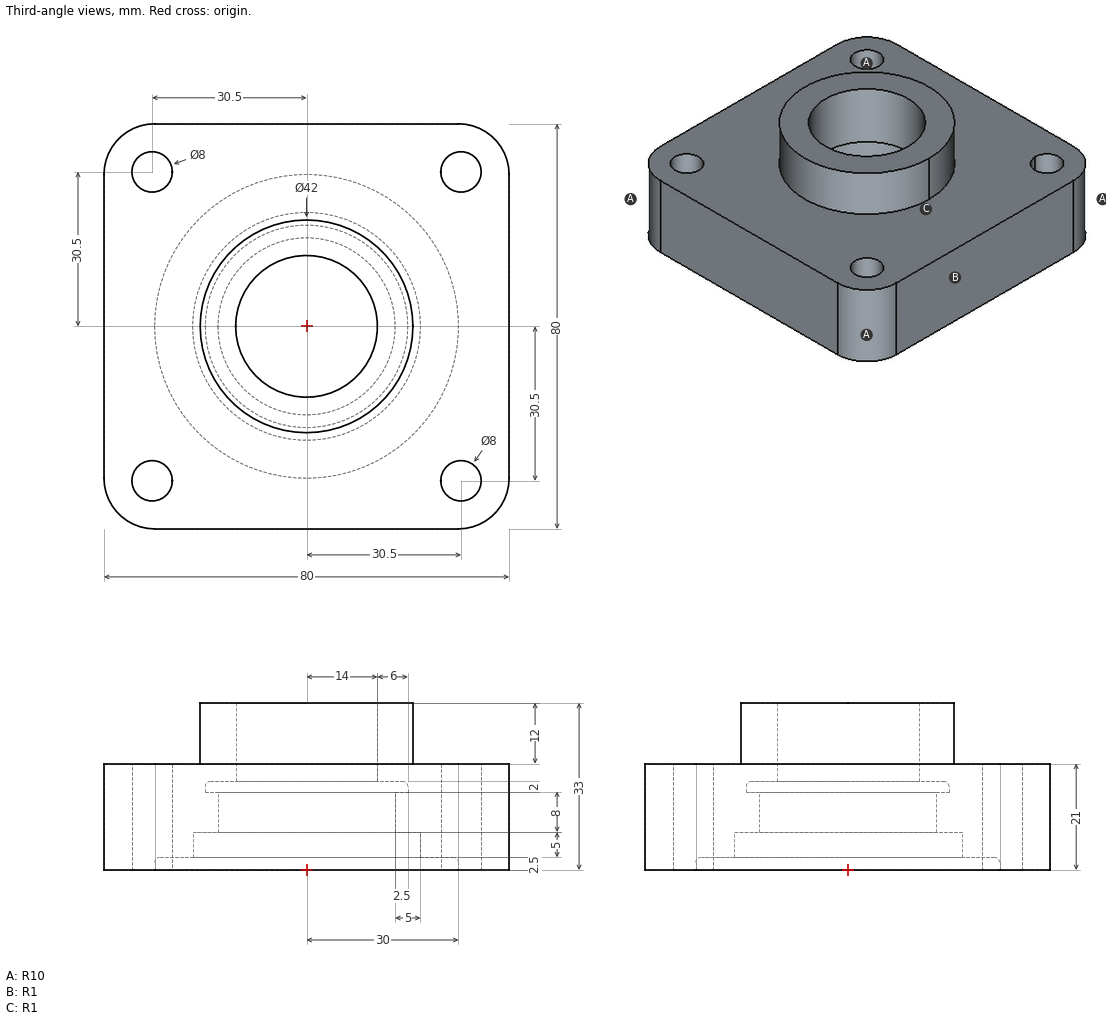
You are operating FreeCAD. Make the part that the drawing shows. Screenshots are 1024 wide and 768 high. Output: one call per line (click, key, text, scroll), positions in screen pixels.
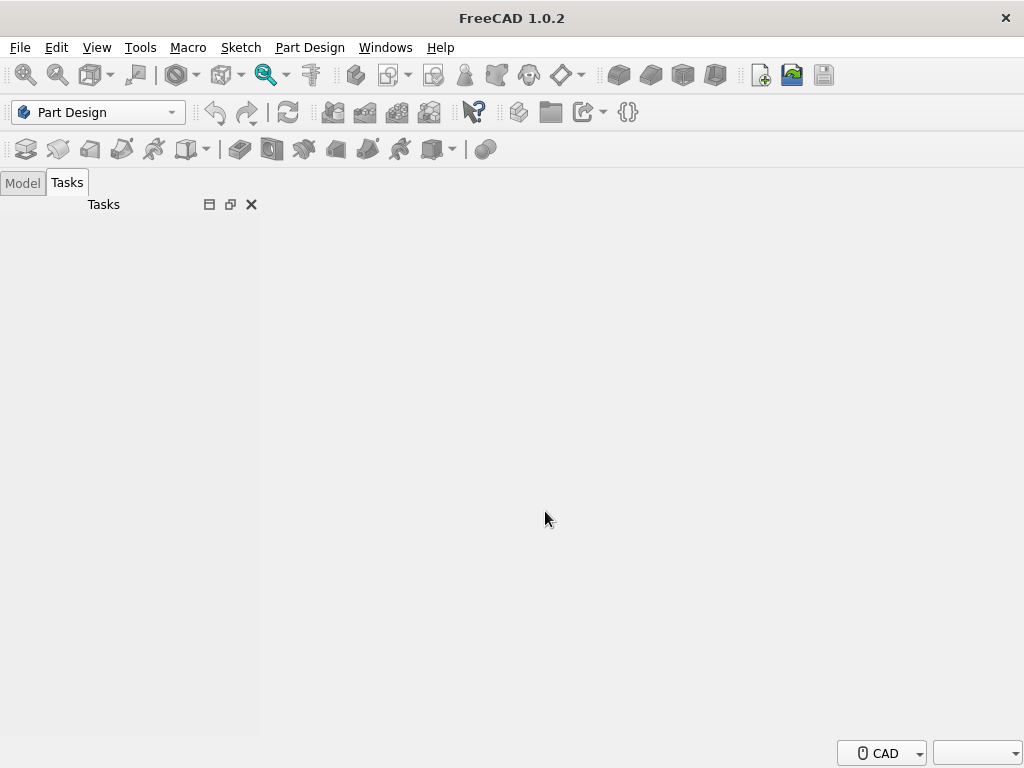
click(760, 76)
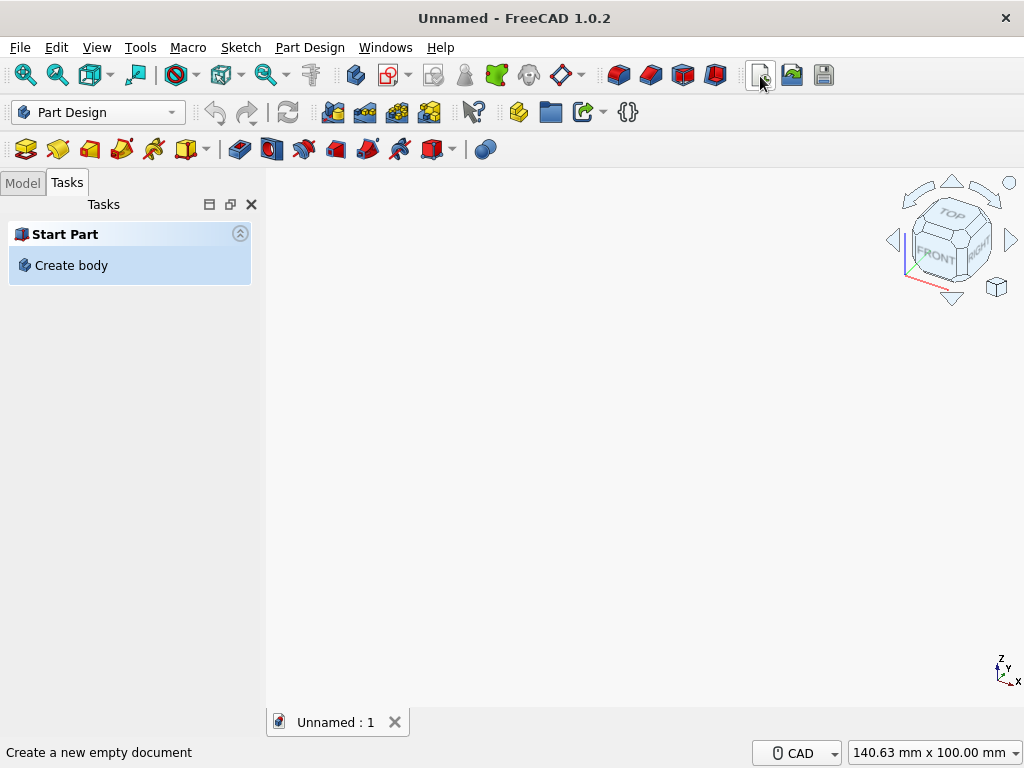
click(388, 76)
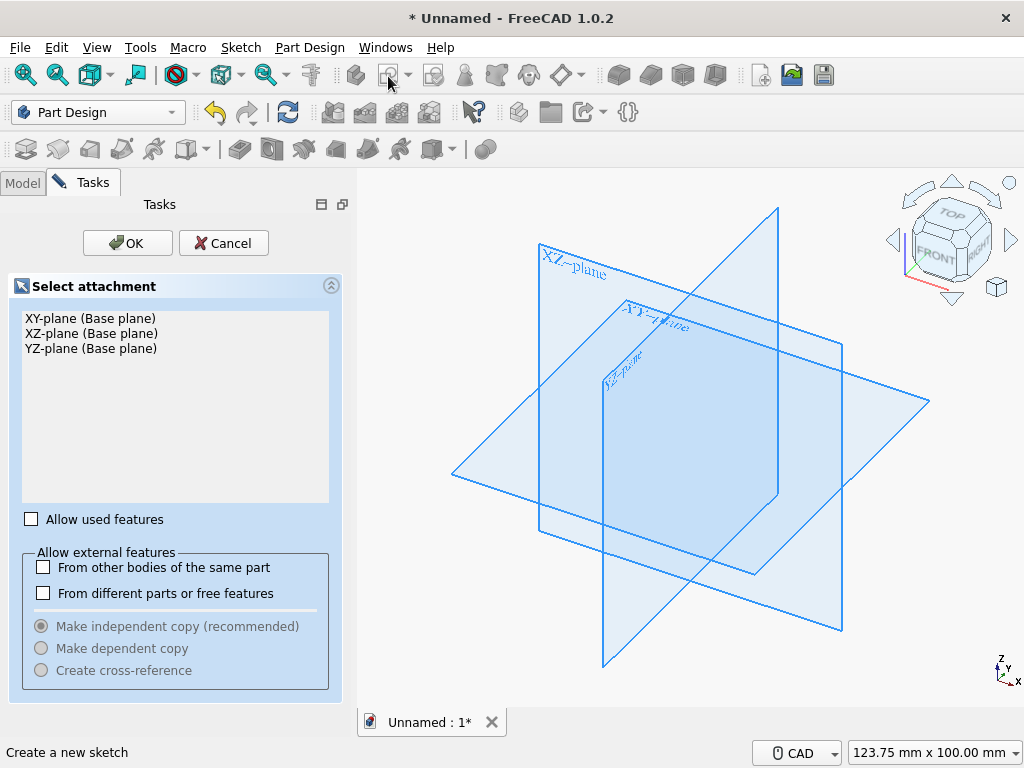
click(82, 318)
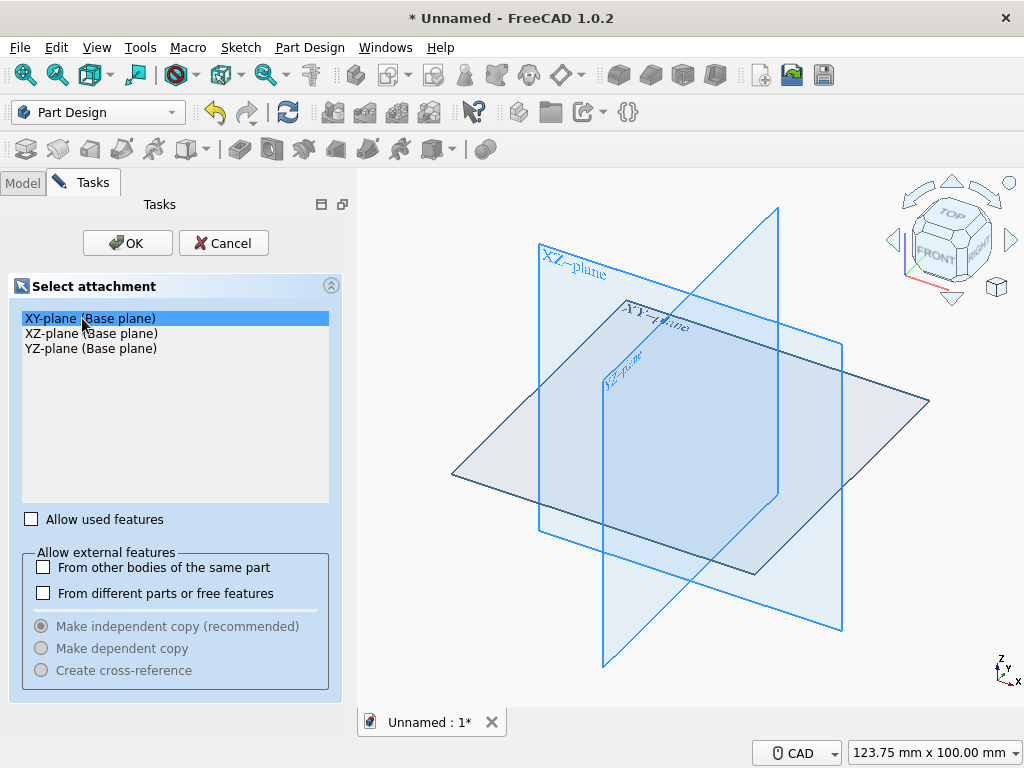
click(128, 243)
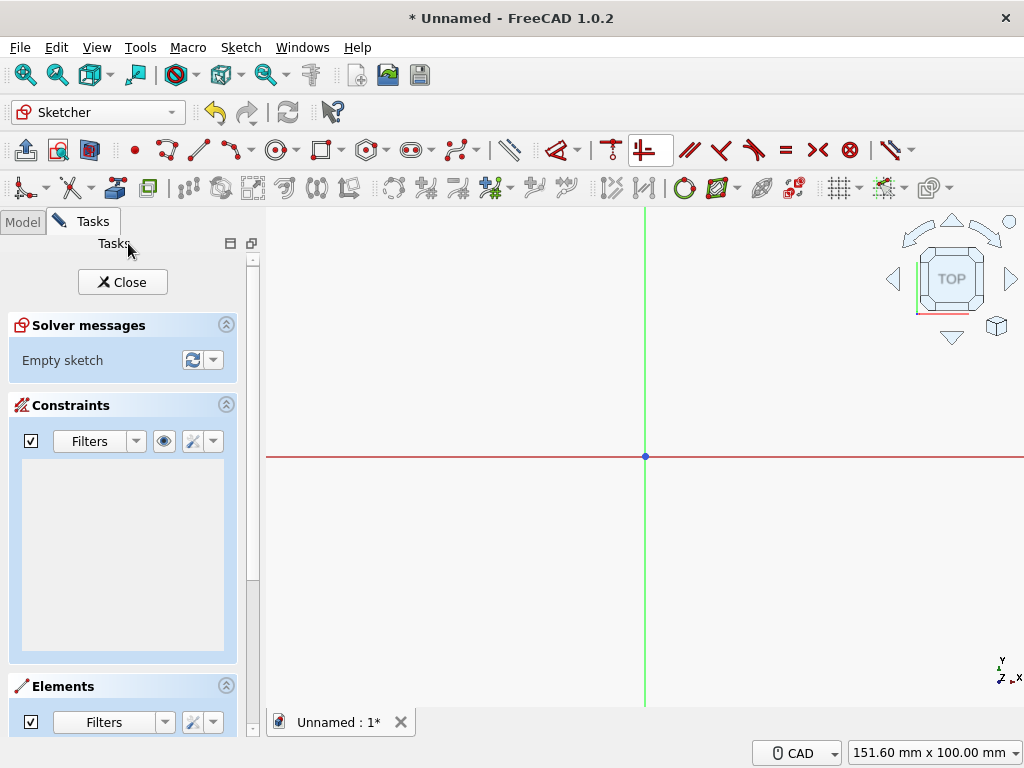
scroll(294, 457, down, 1)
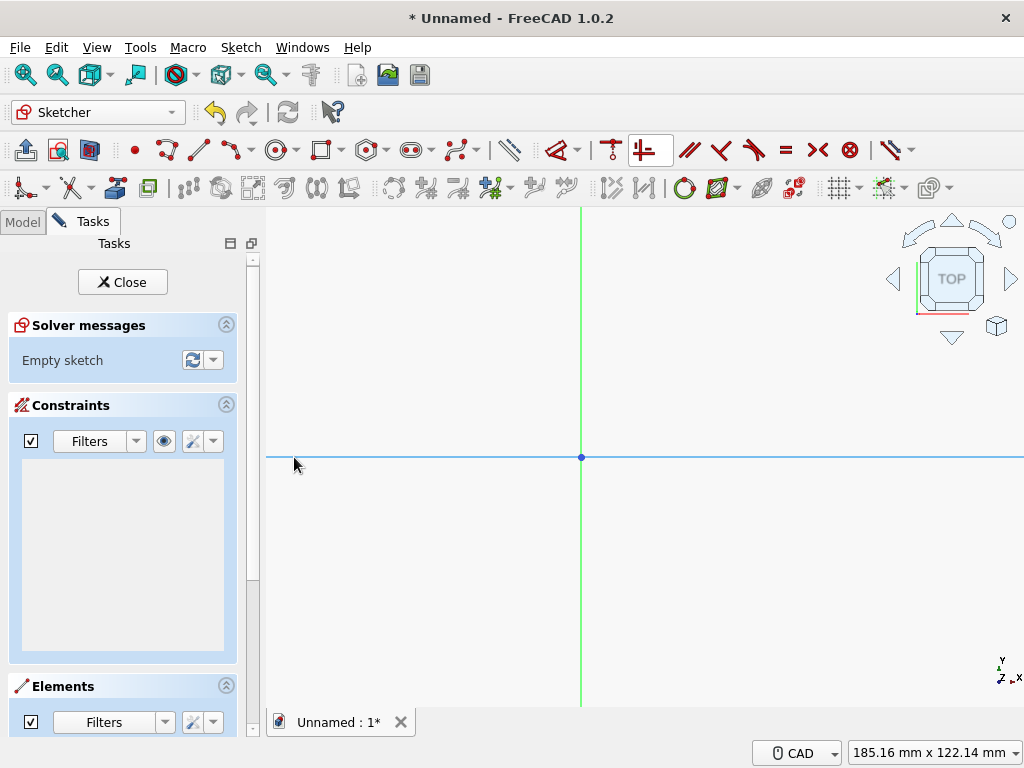
key(g)
key(v)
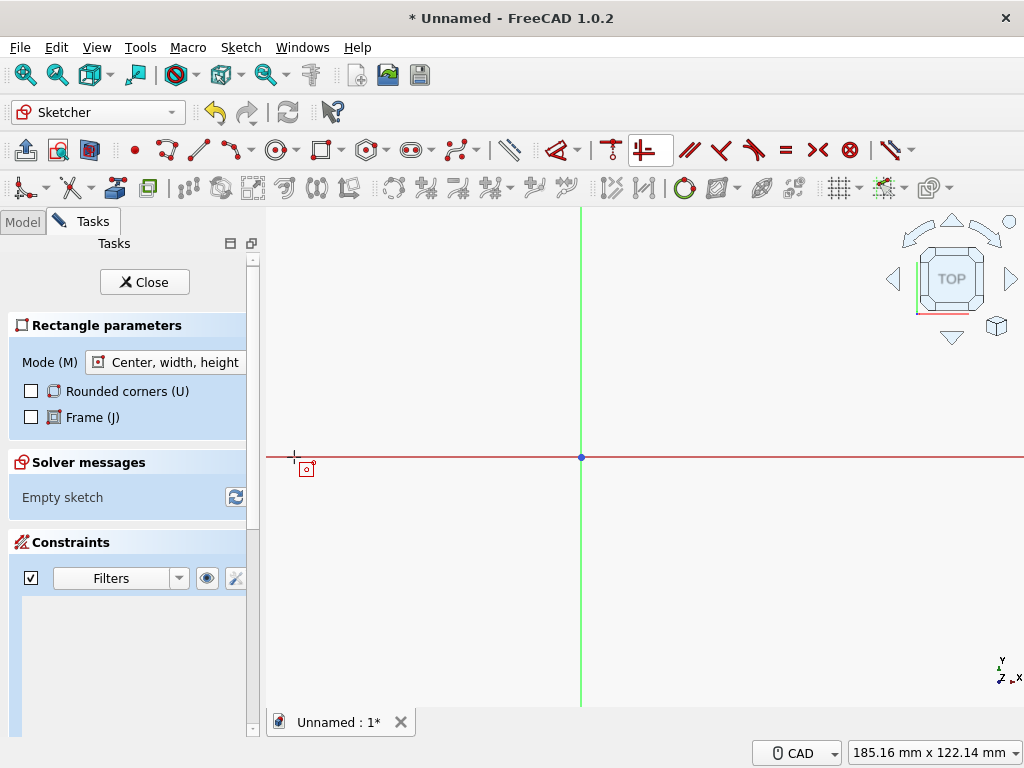
click(581, 457)
move(745, 293)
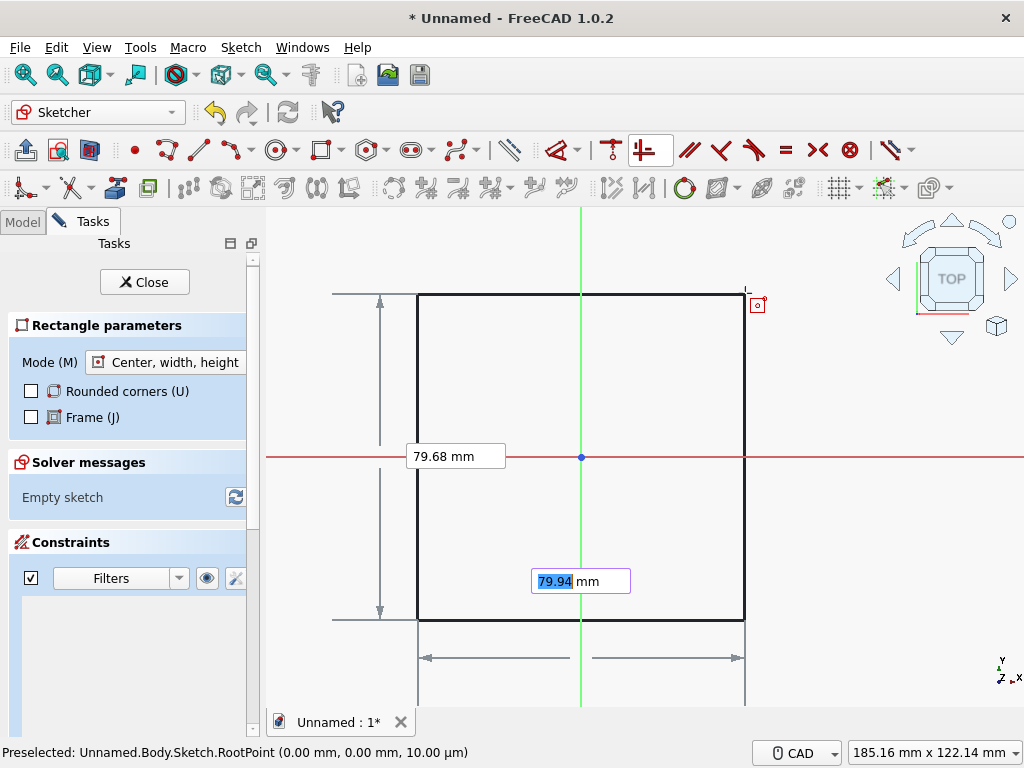
text(80)
key(Tab)
text(80)
key(Return)
key(Escape)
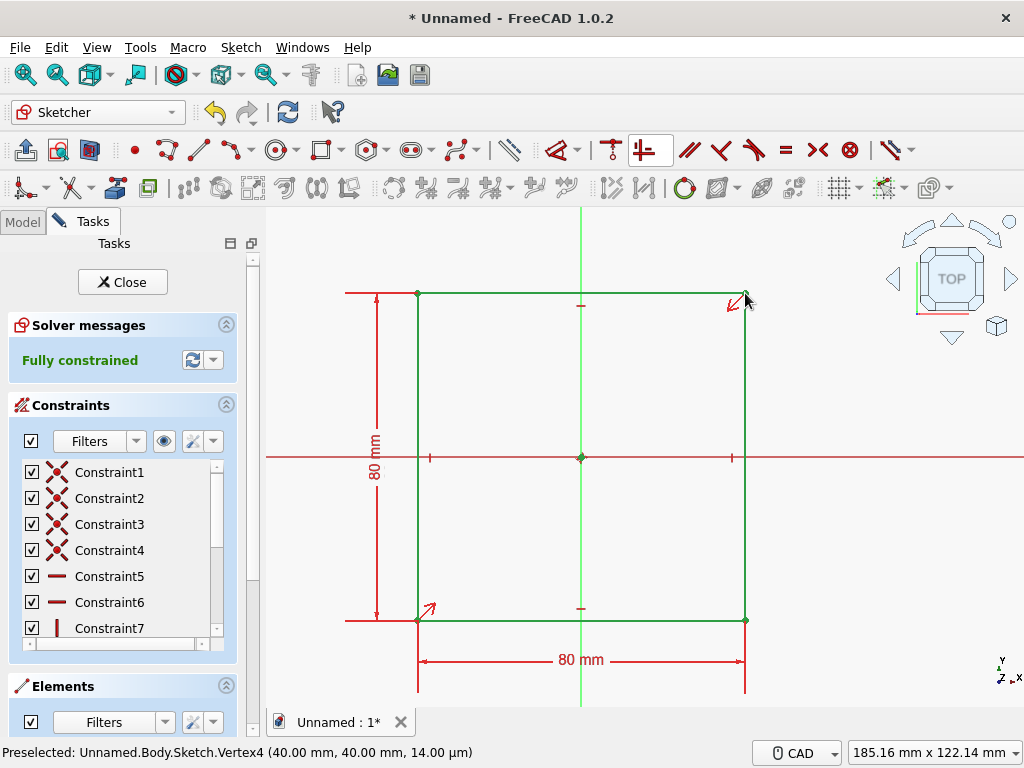
click(123, 282)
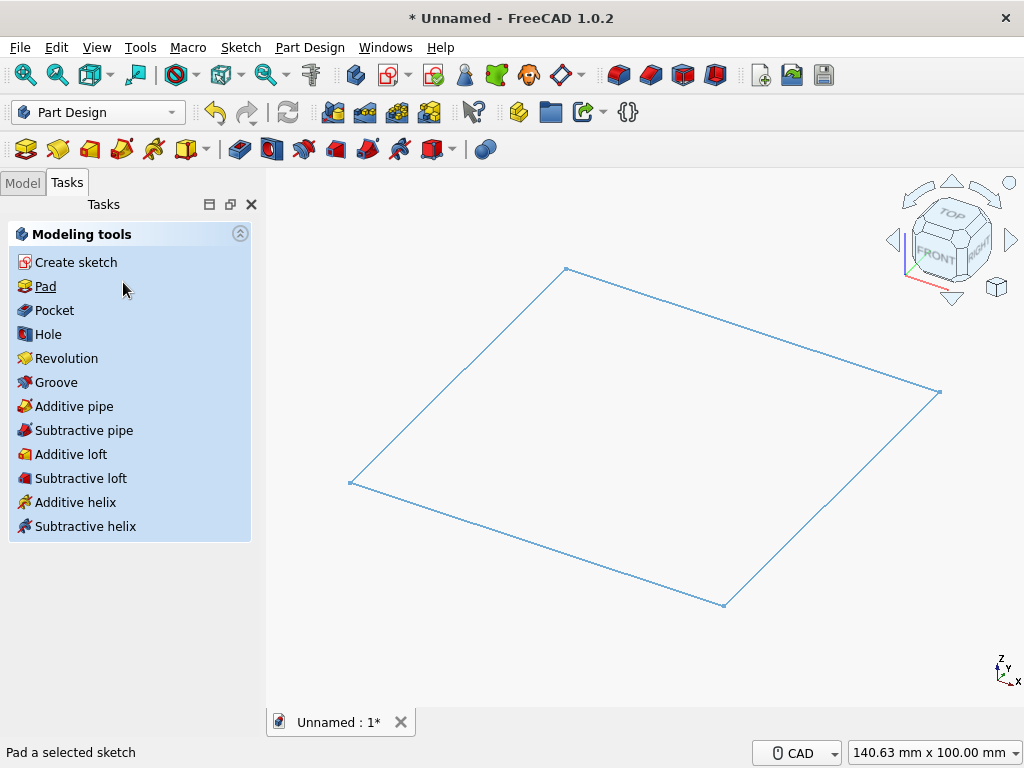
click(26, 150)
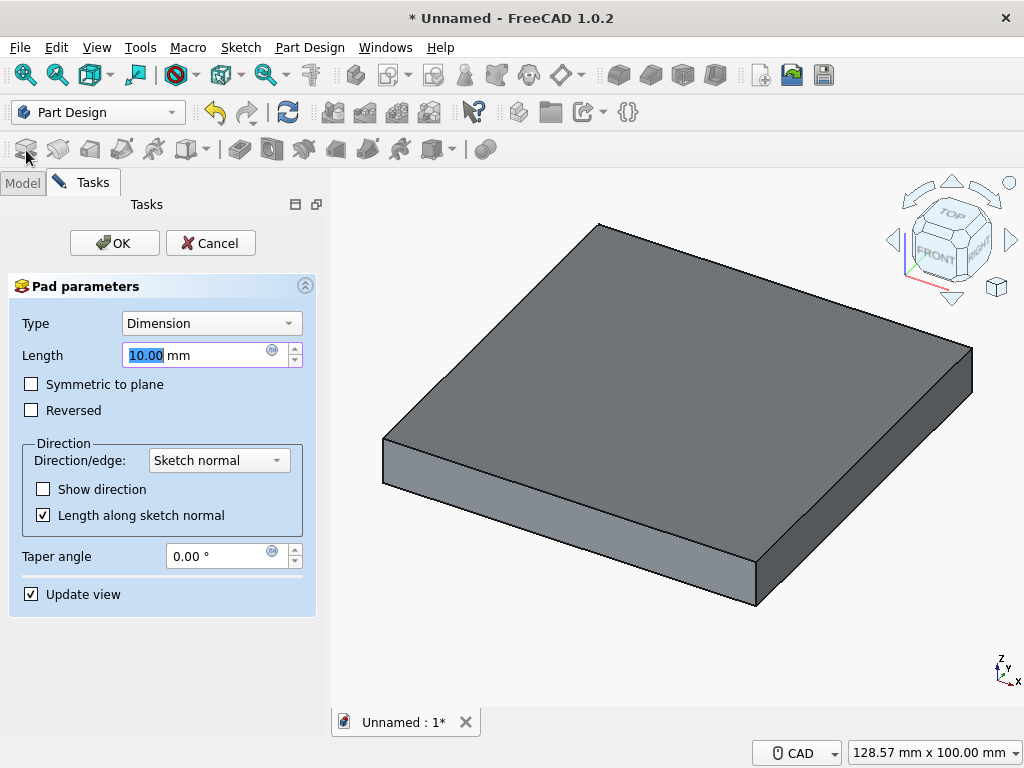
text(21)
key(Tab)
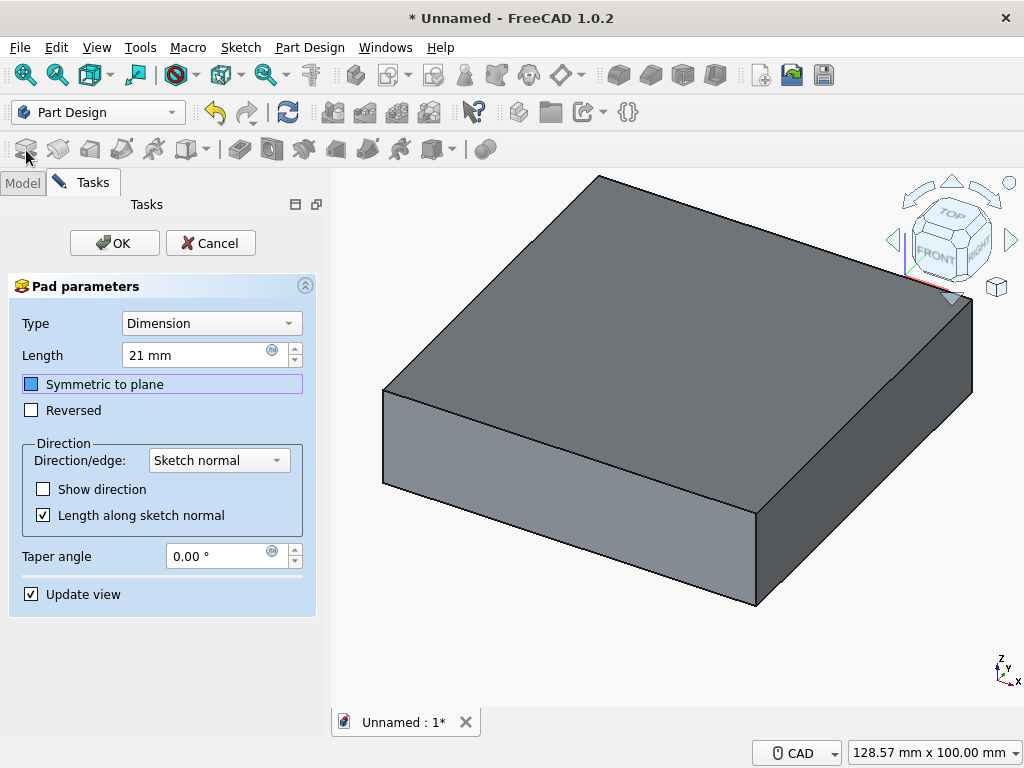
click(115, 243)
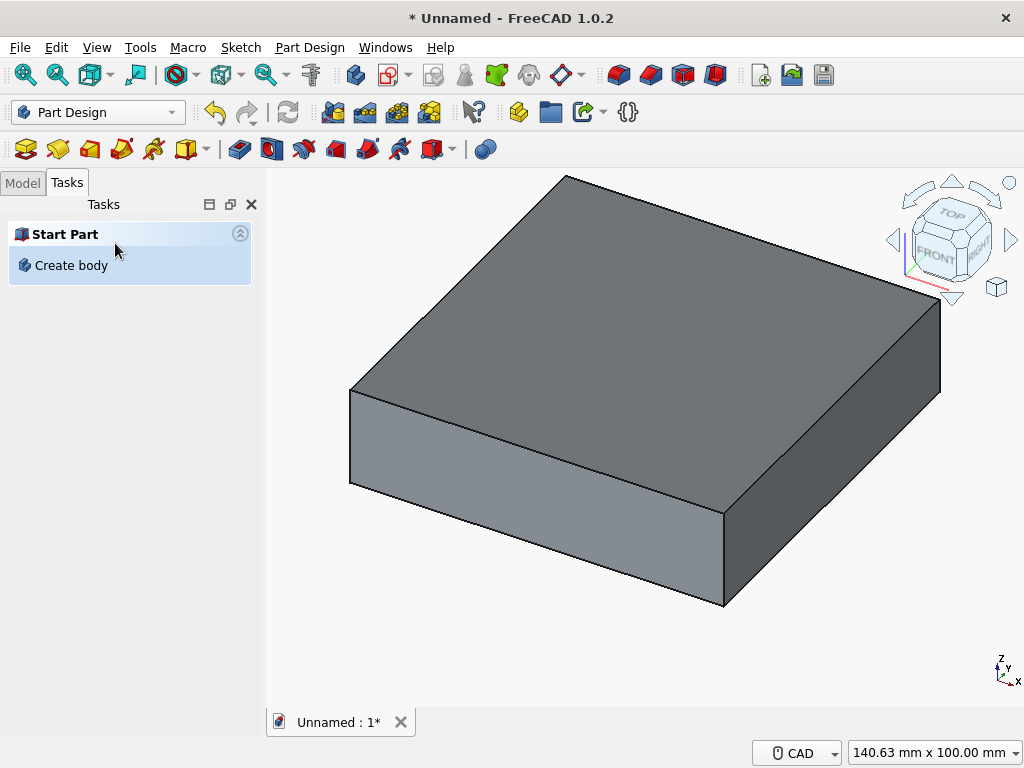
click(645, 344)